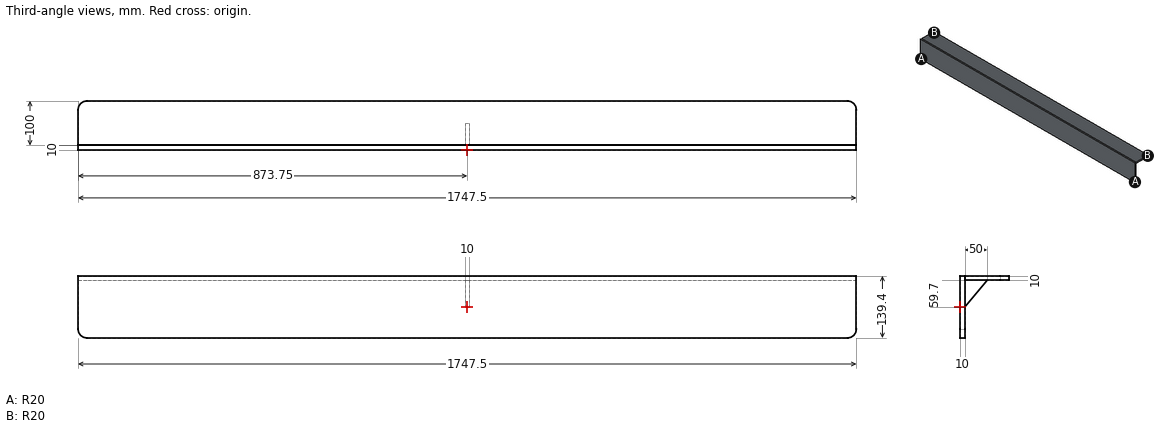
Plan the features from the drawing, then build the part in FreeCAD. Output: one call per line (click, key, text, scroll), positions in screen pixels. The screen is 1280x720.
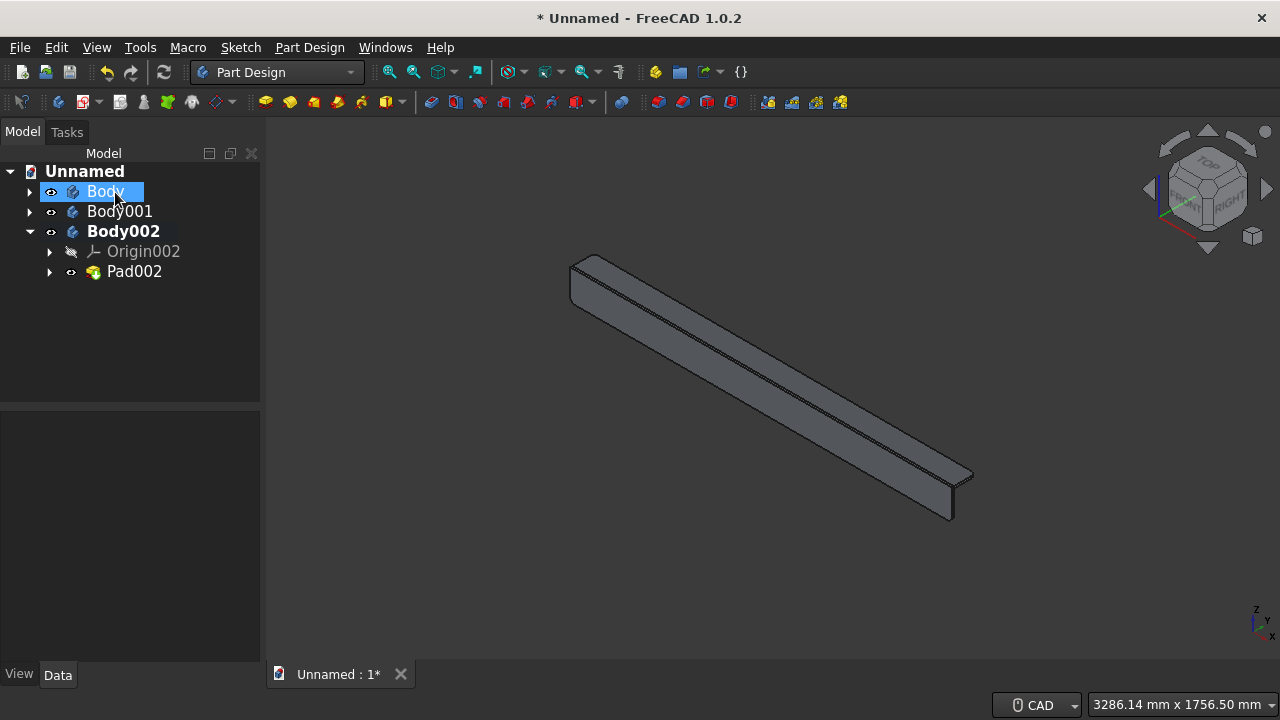
click(390, 72)